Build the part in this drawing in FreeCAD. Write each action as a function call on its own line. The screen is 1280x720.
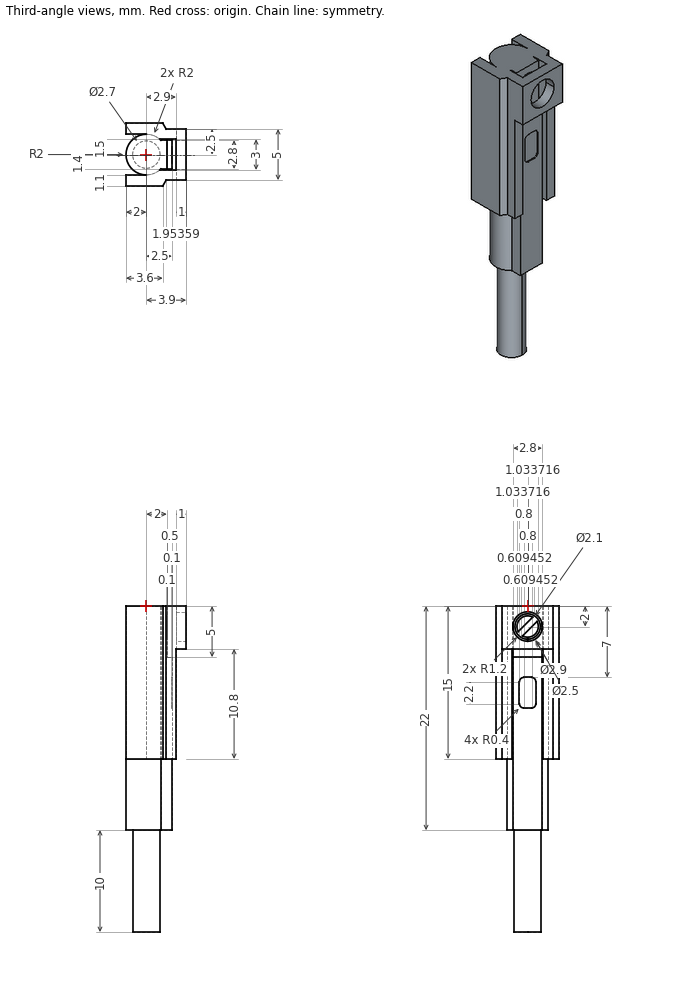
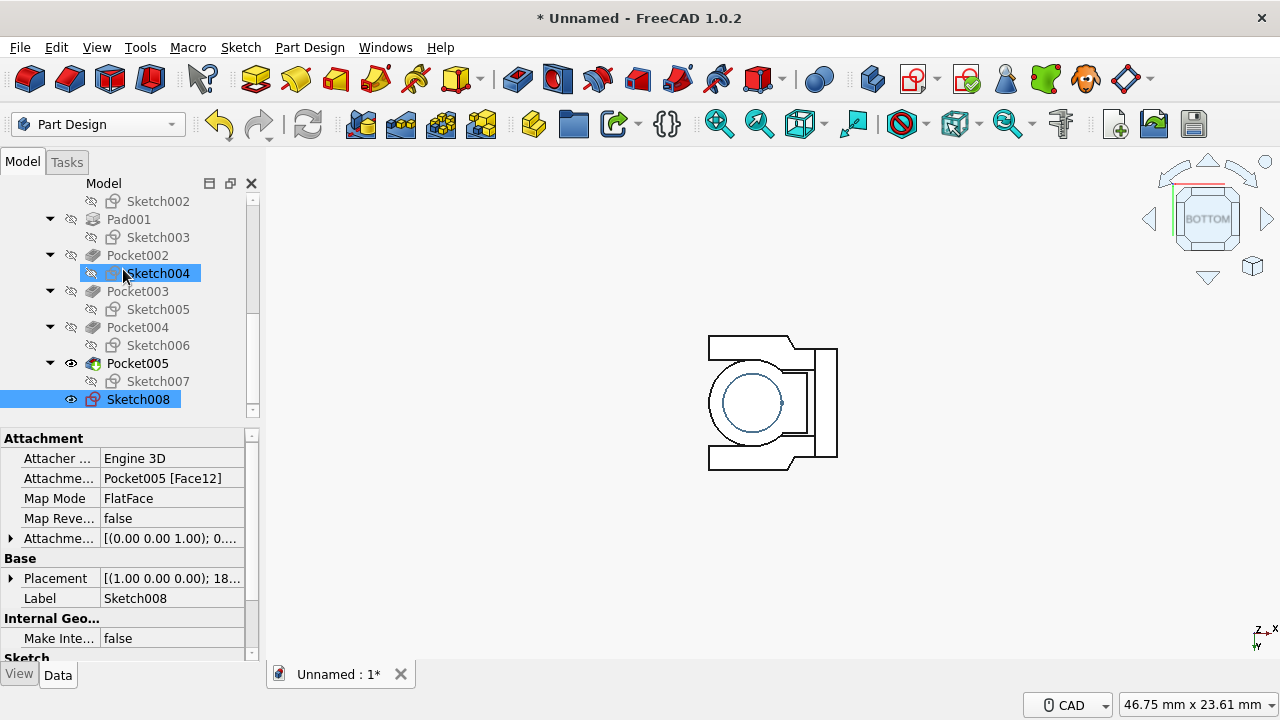
click(256, 80)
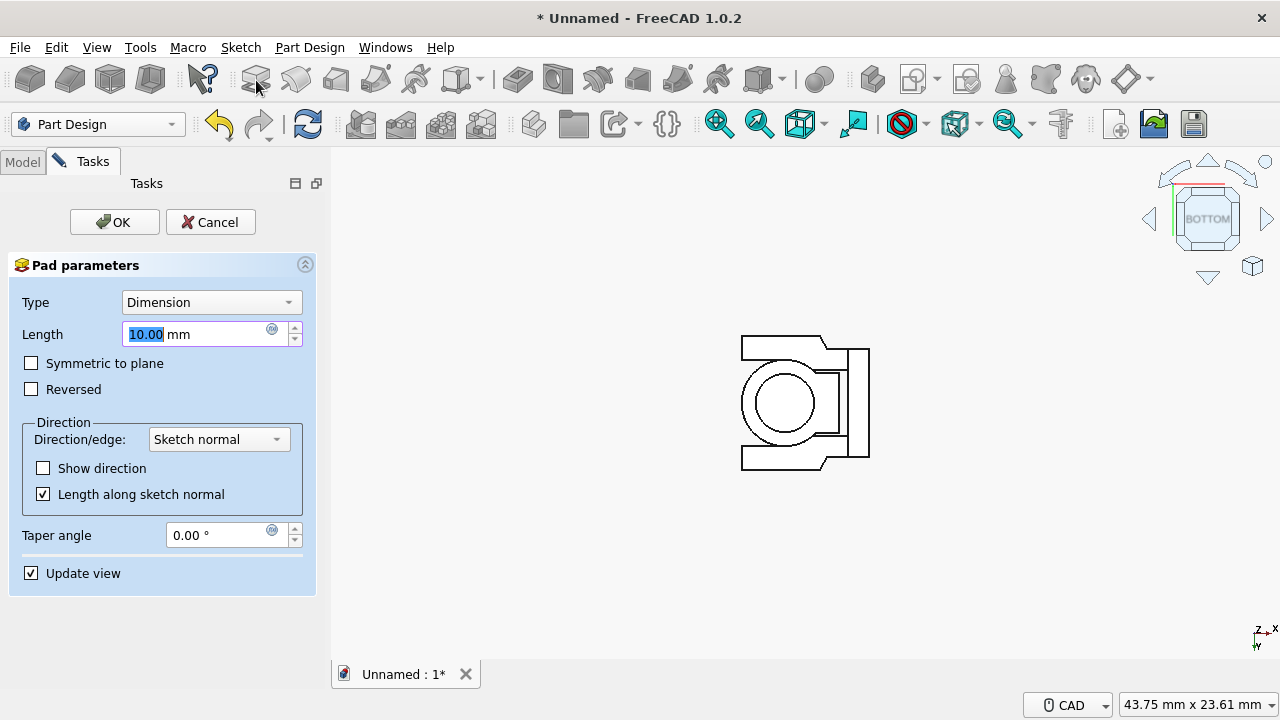
text(10)
key(Tab)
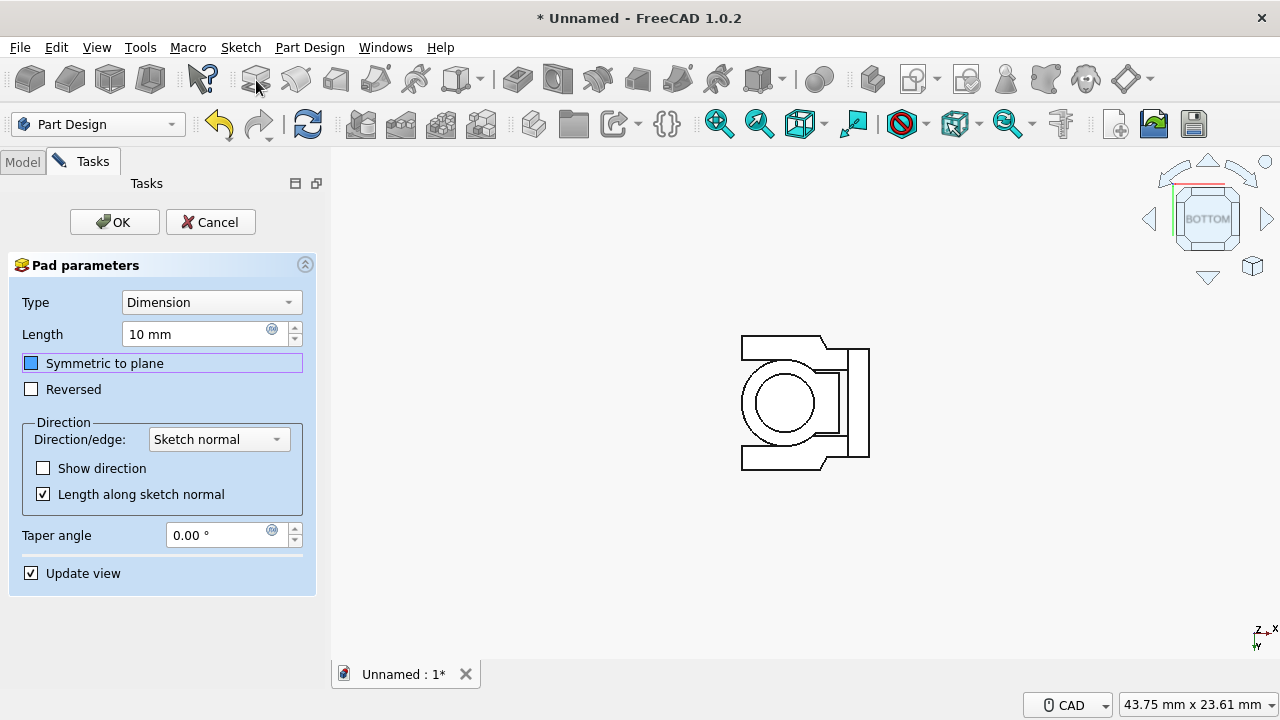
click(115, 222)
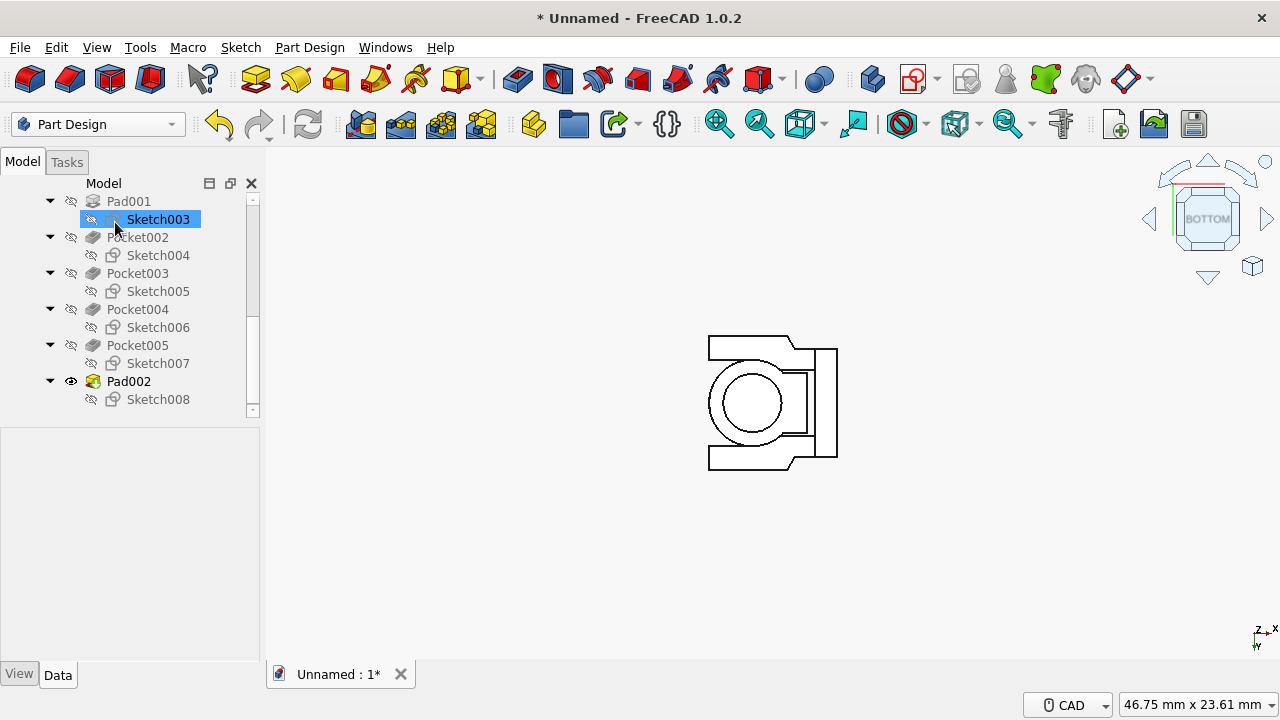
key(0)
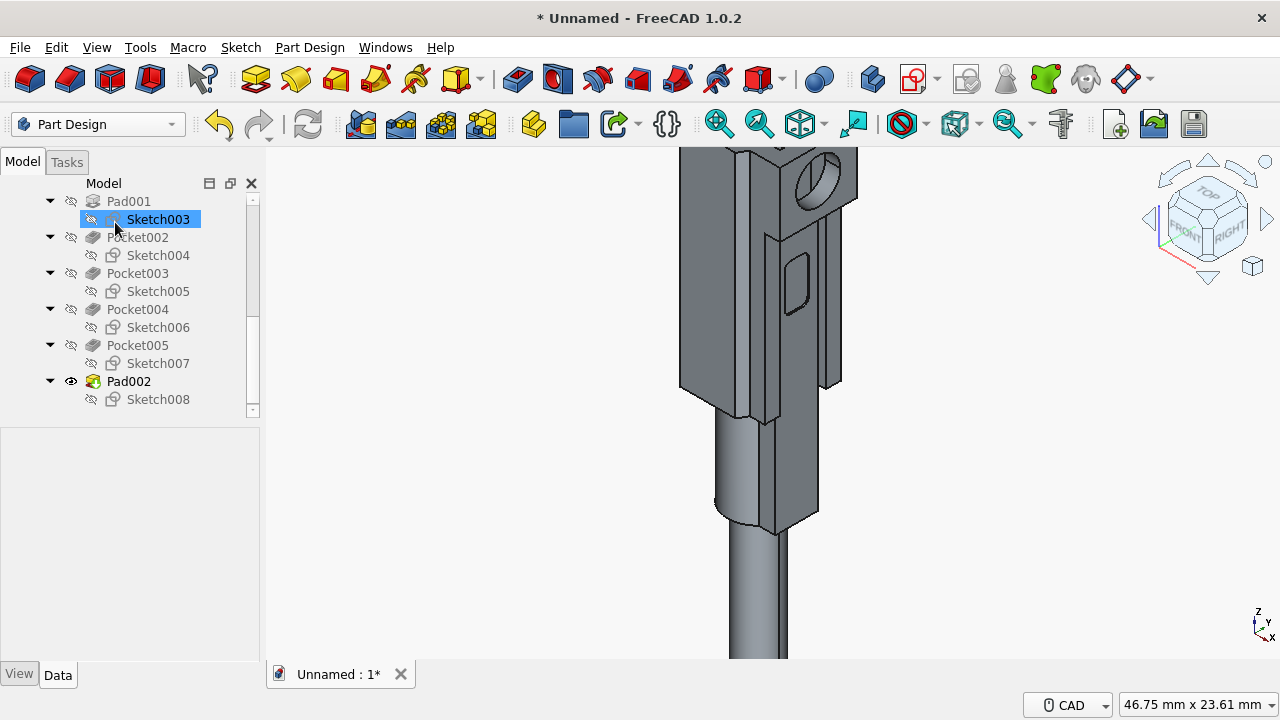
click(720, 124)